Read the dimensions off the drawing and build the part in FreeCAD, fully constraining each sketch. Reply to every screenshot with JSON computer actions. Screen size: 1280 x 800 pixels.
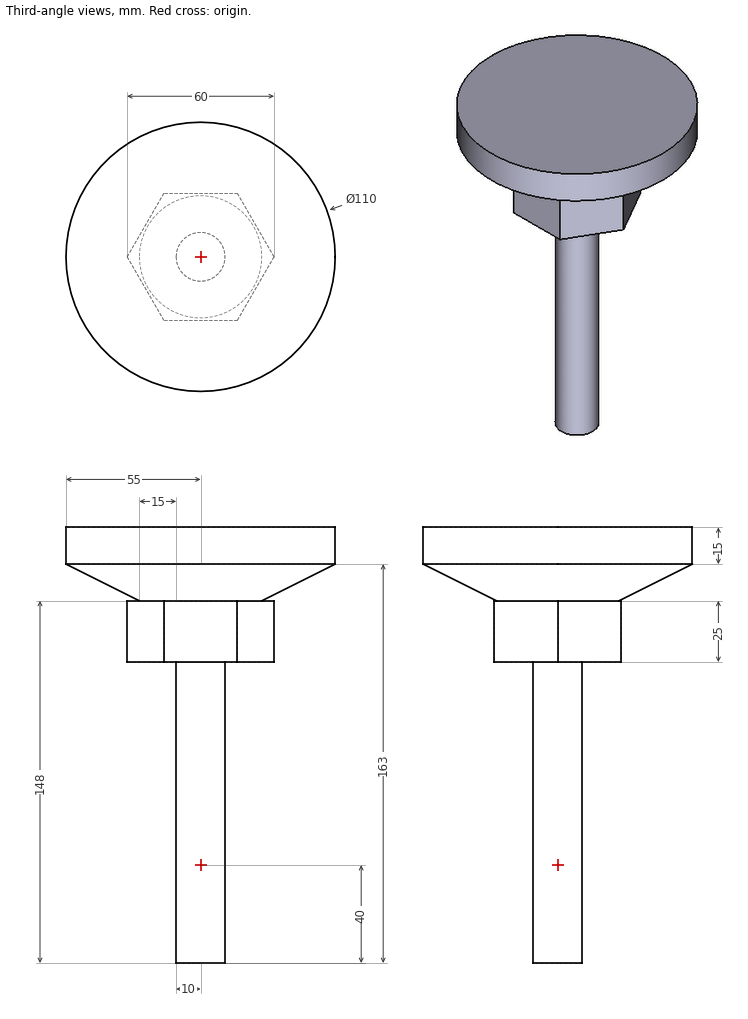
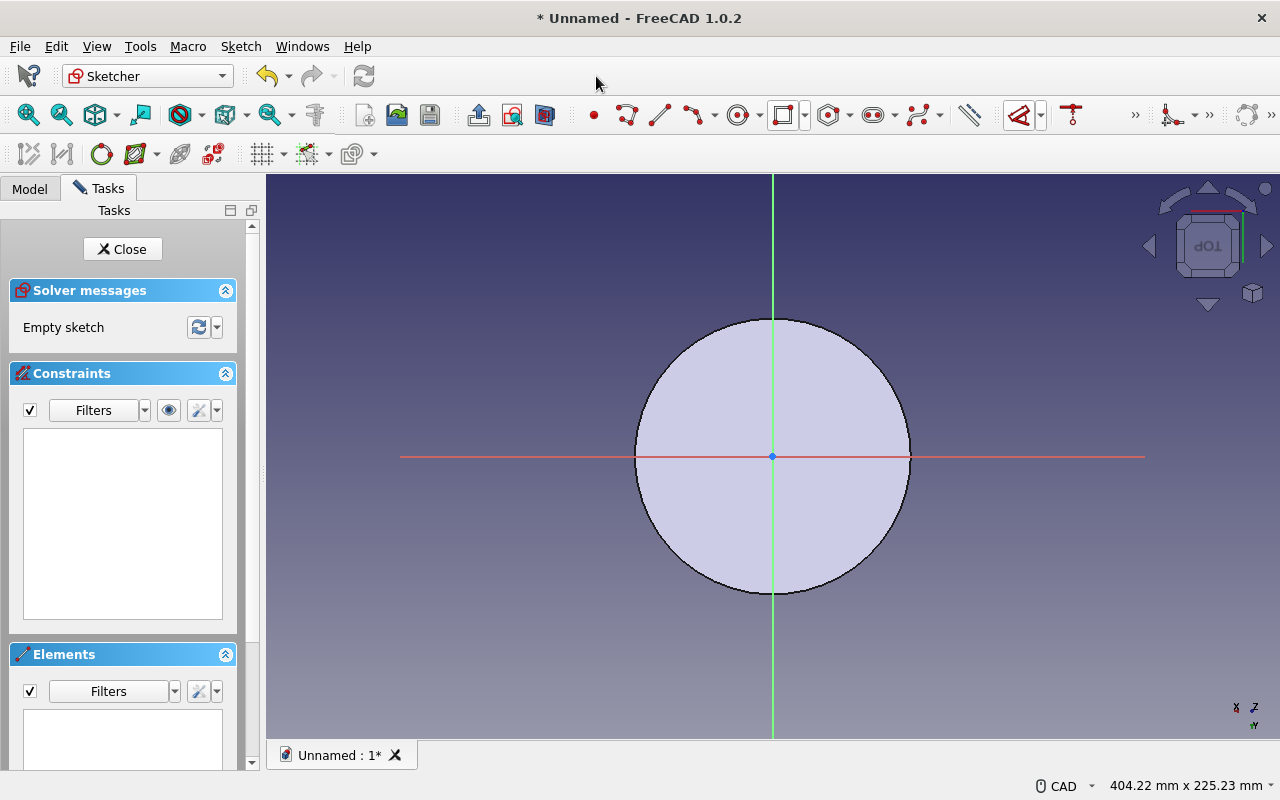
{"action": "left_click", "coordinate": [738, 116]}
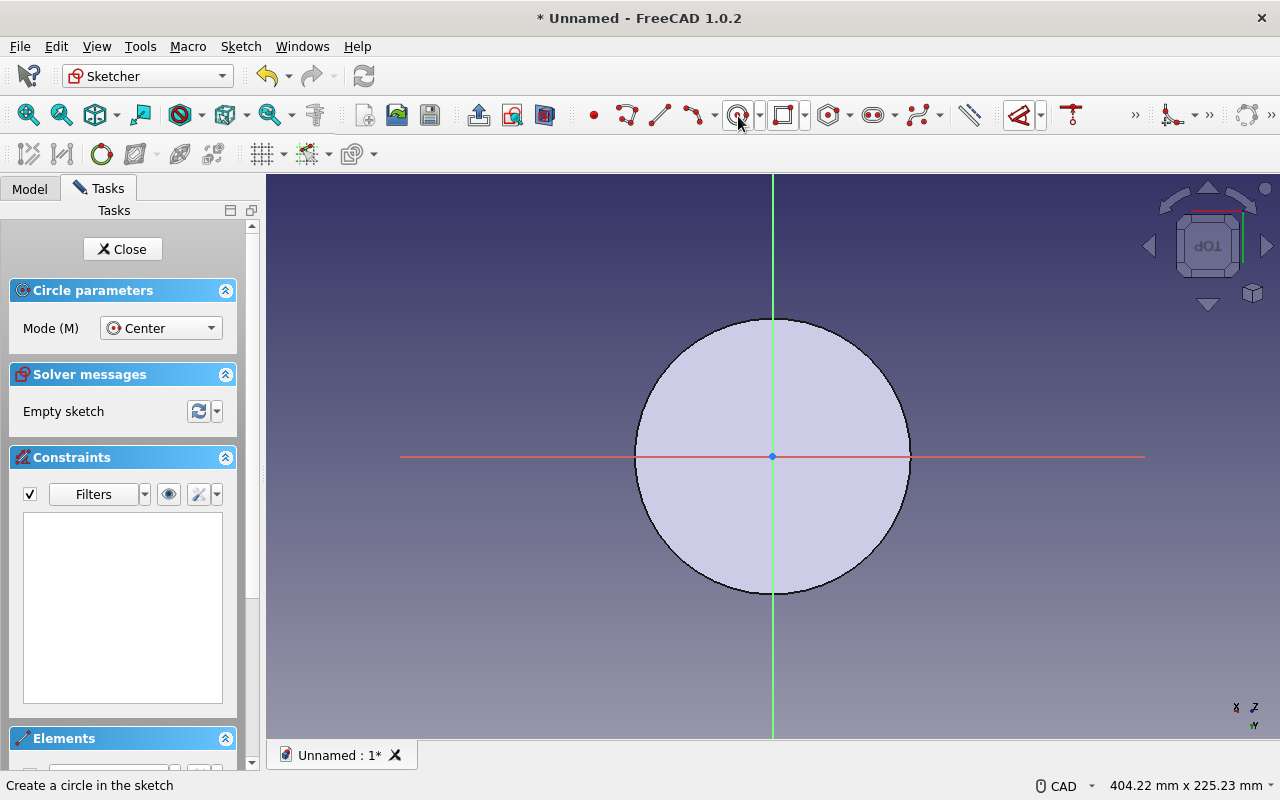
{"action": "left_click", "coordinate": [773, 457]}
{"action": "mouse_move", "coordinate": [870, 359]}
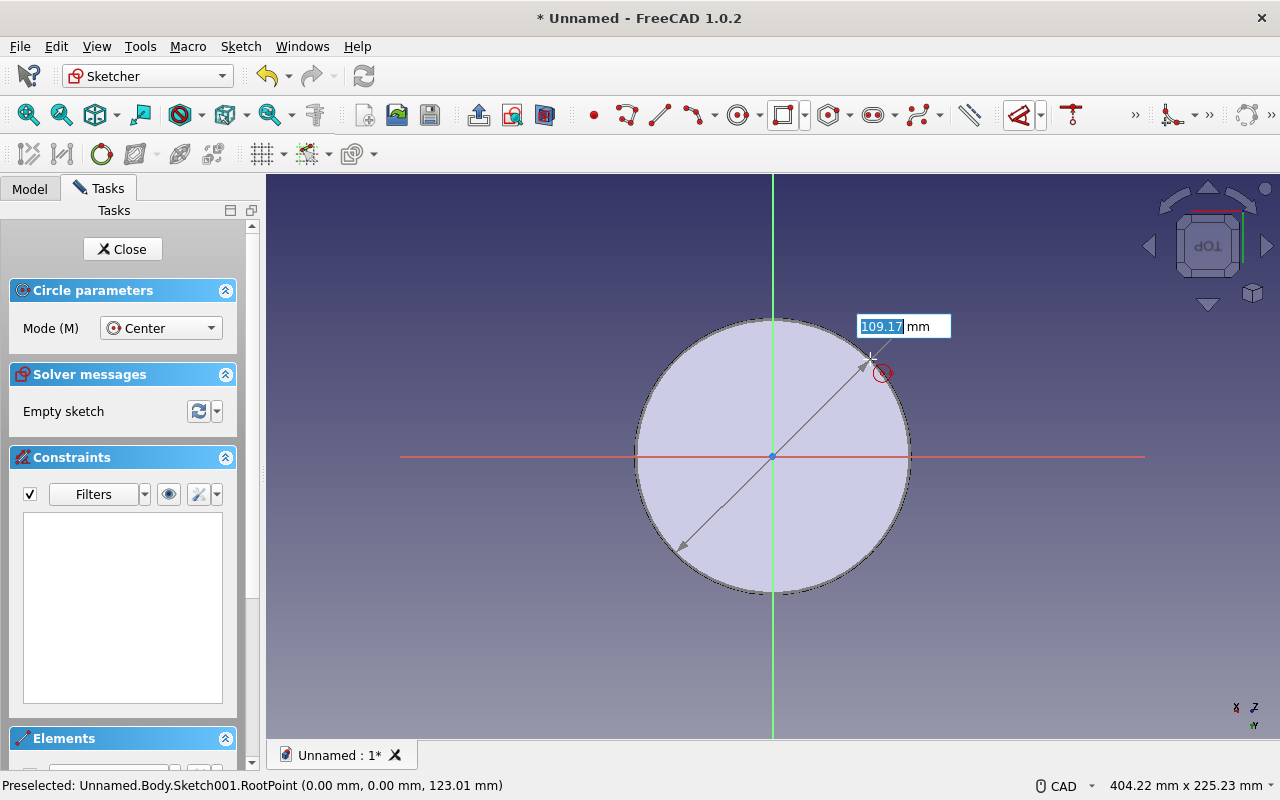
{"action": "type", "text": "110"}
{"action": "key", "text": "Return"}
{"action": "key", "text": "Escape"}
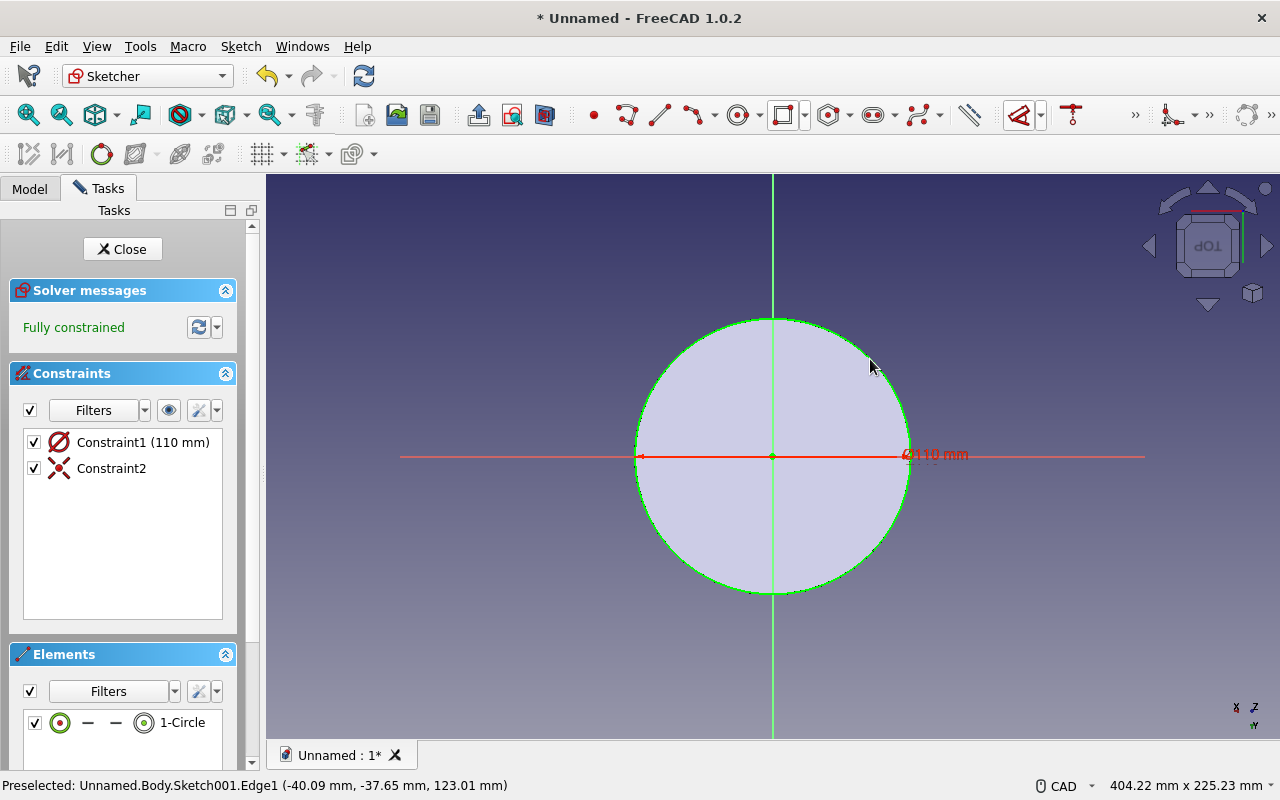
{"action": "left_click", "coordinate": [123, 249]}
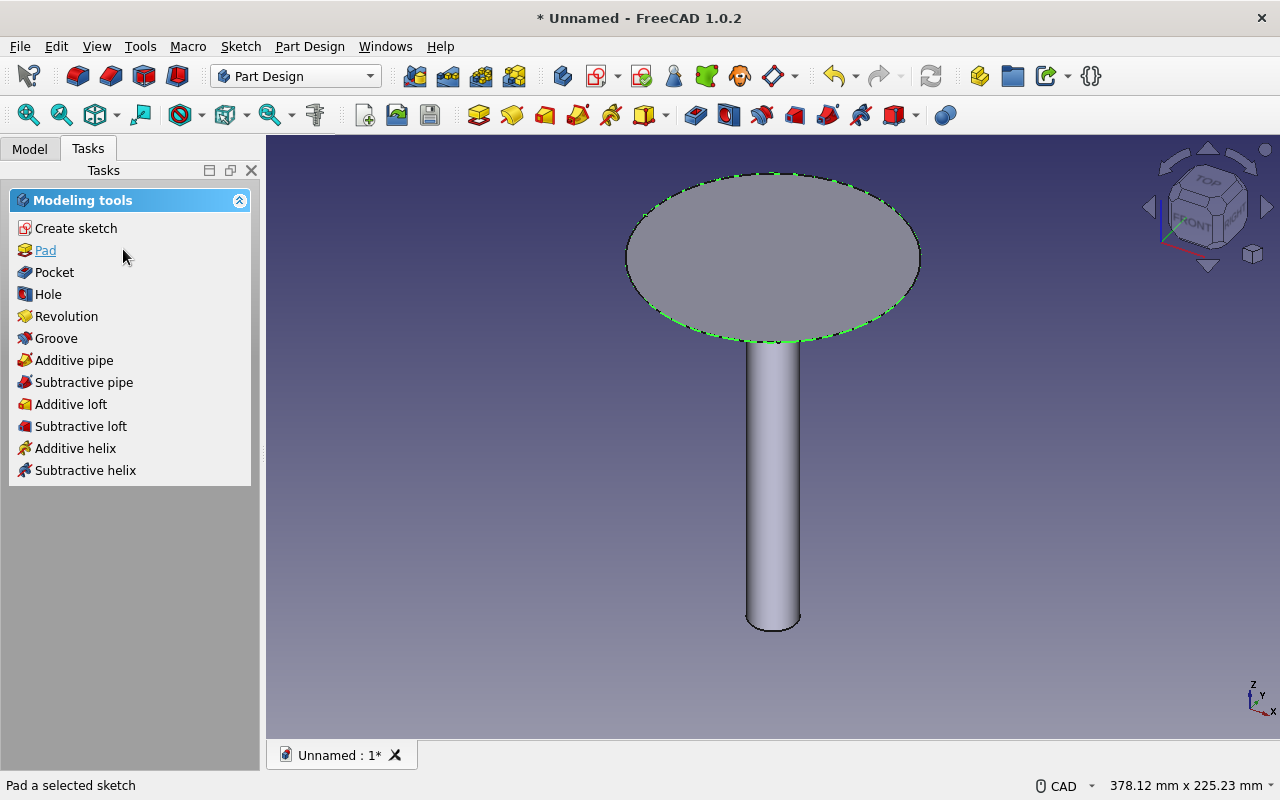
{"action": "left_click", "coordinate": [479, 116]}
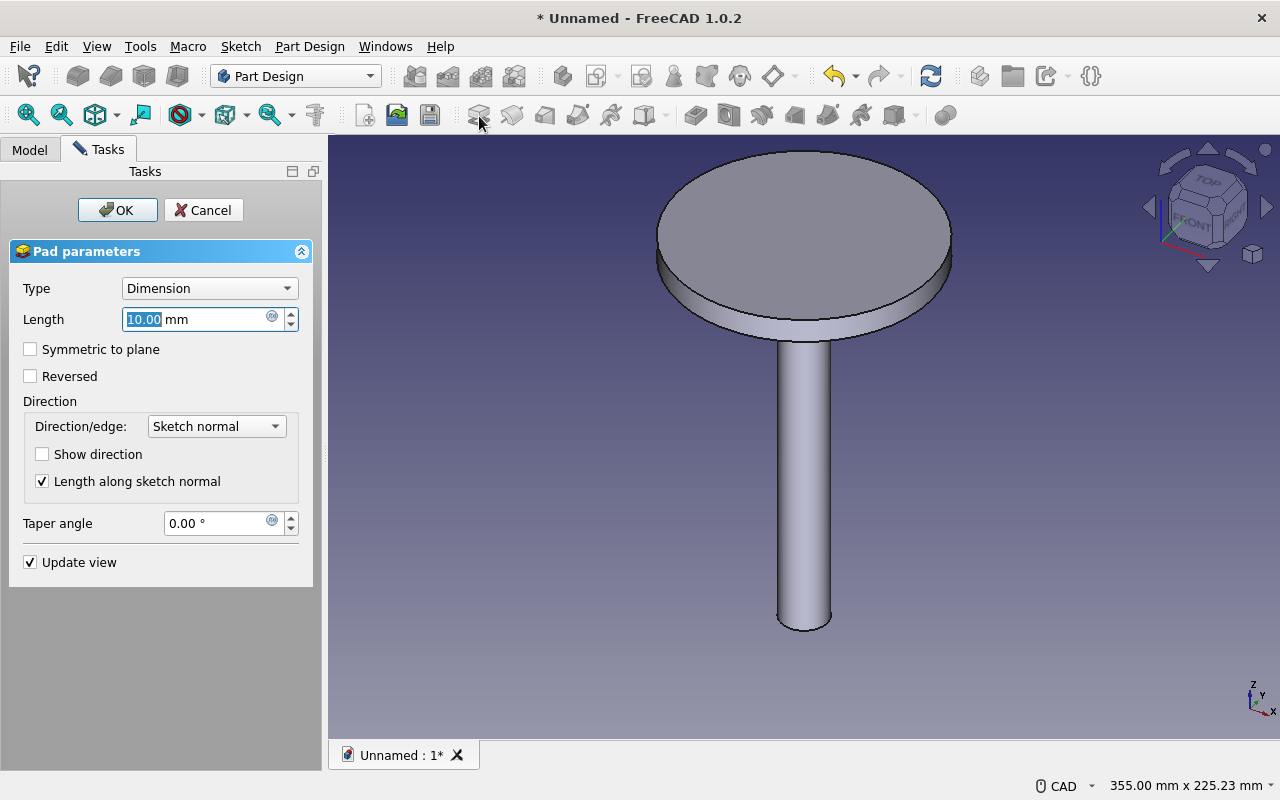
{"action": "type", "text": "15"}
{"action": "key", "text": "Tab"}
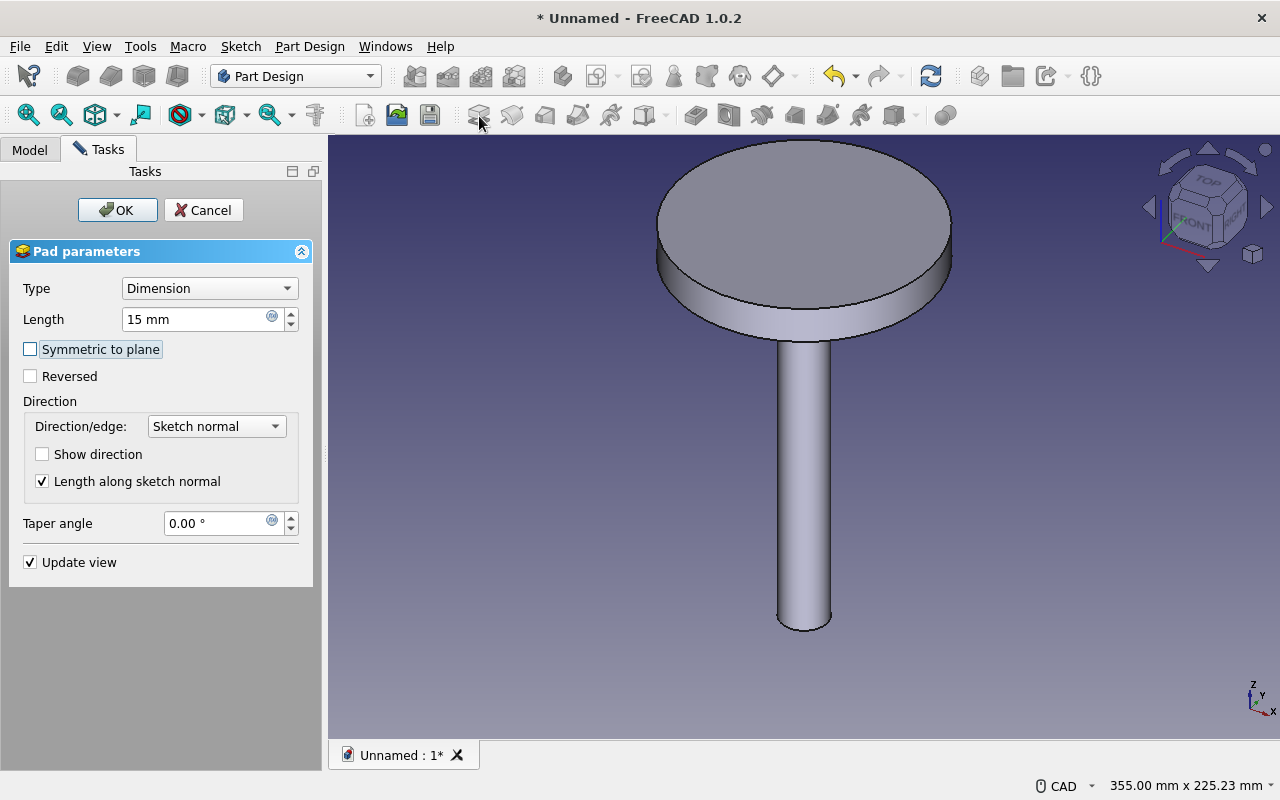
{"action": "left_click", "coordinate": [118, 210]}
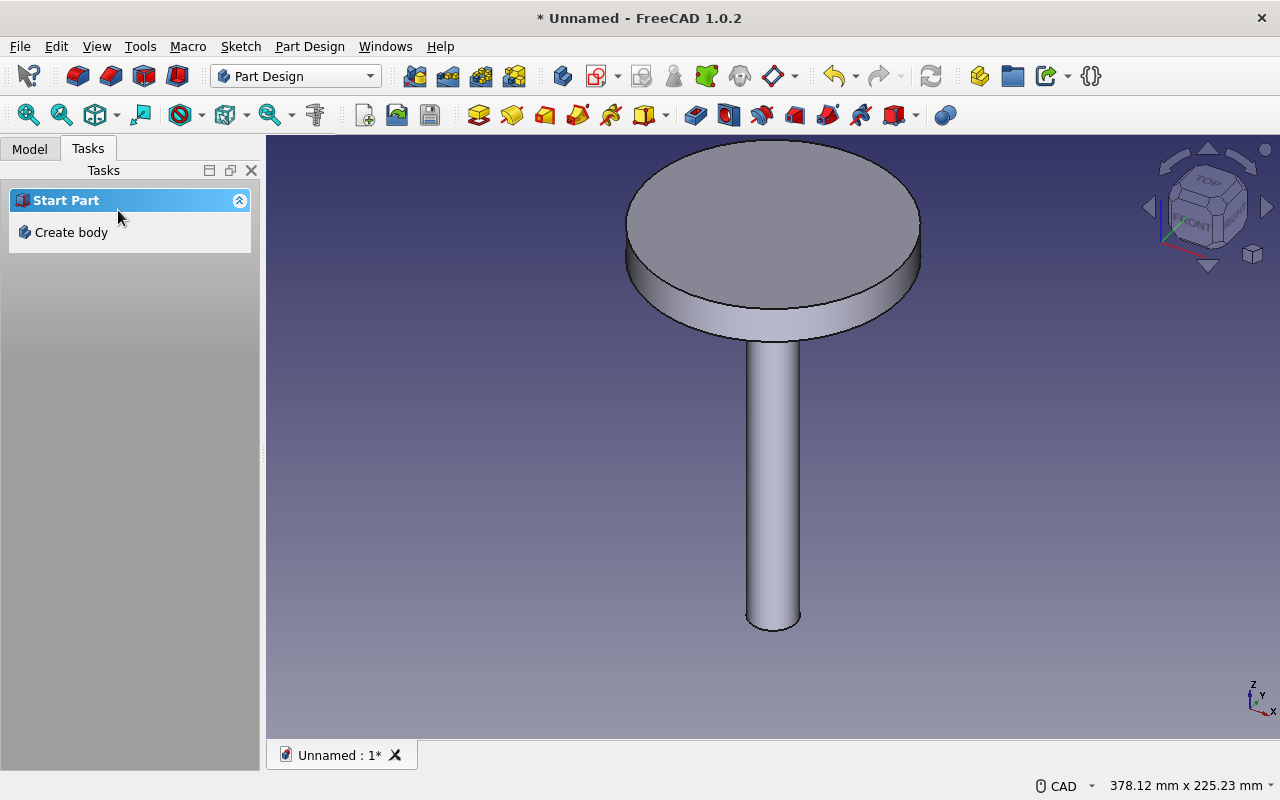
{"action": "left_click", "coordinate": [29, 116]}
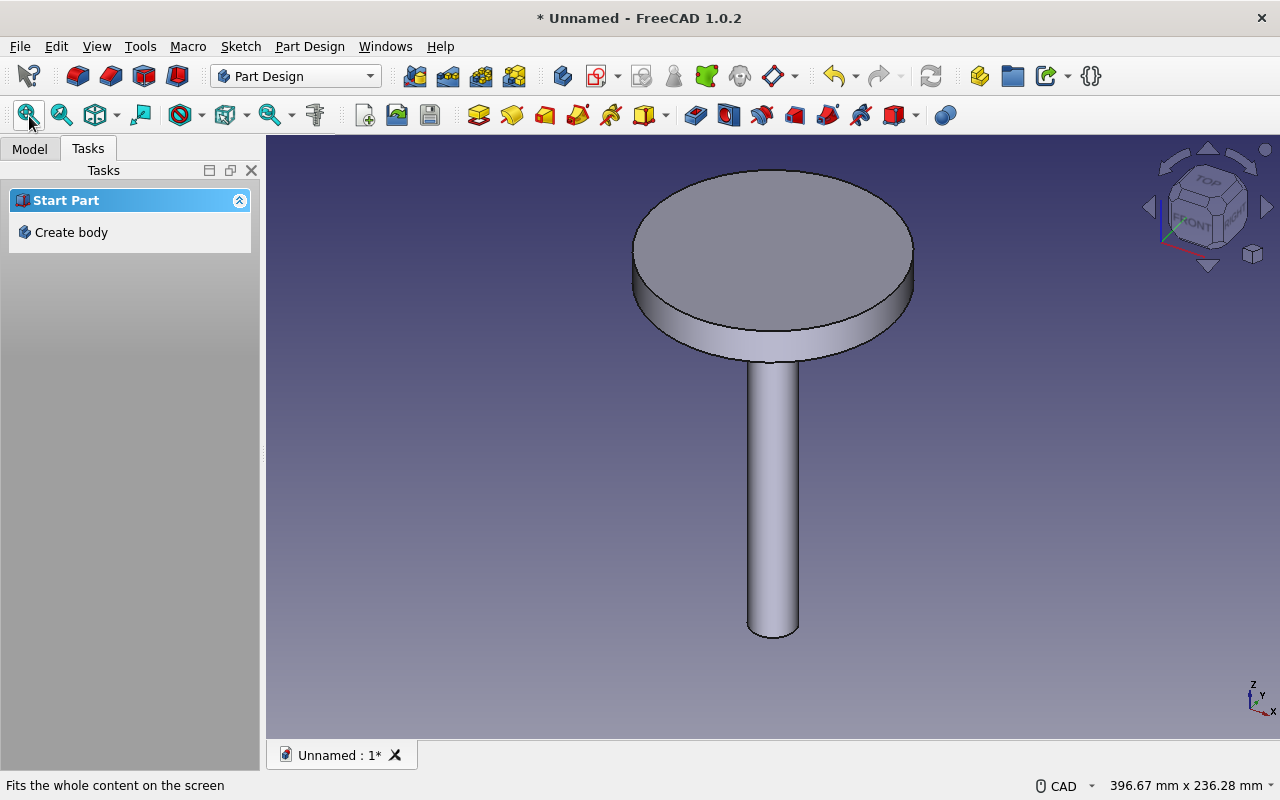
{"action": "key", "text": "5"}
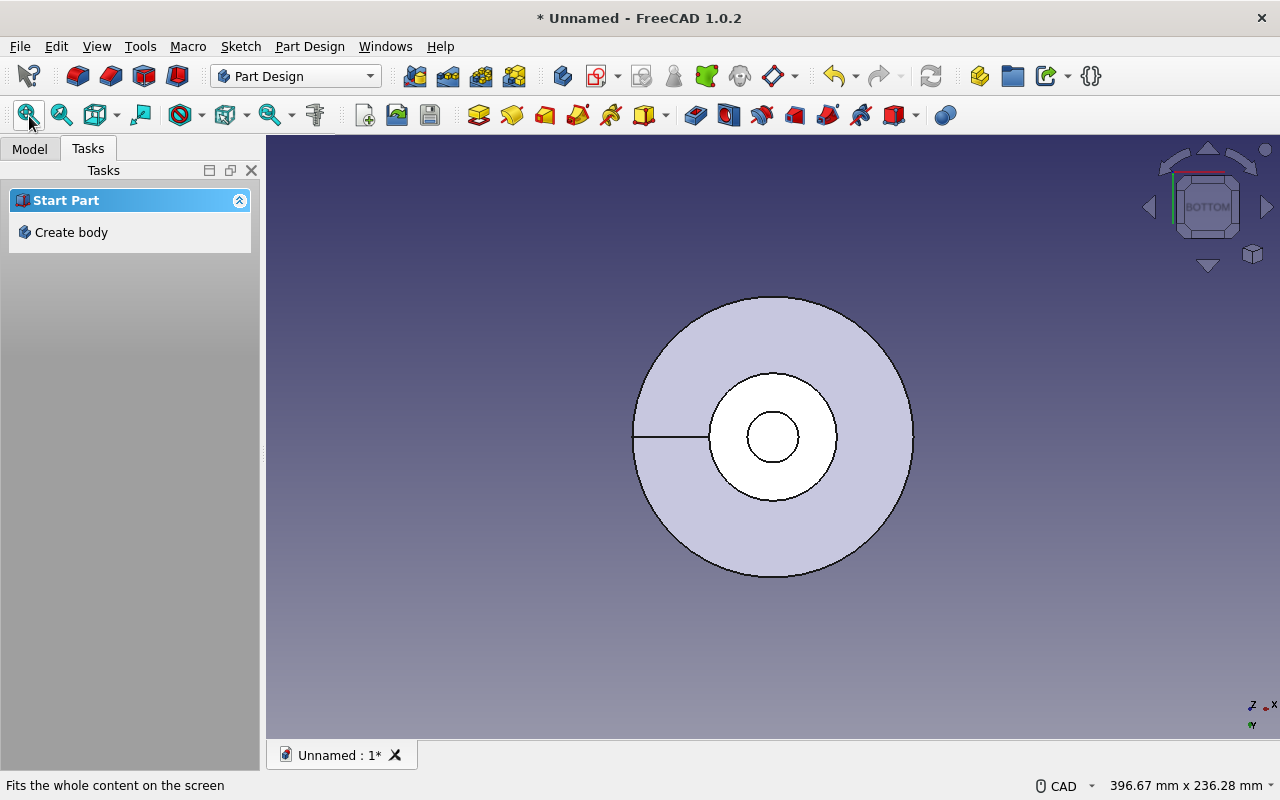
{"action": "left_click", "coordinate": [736, 418]}